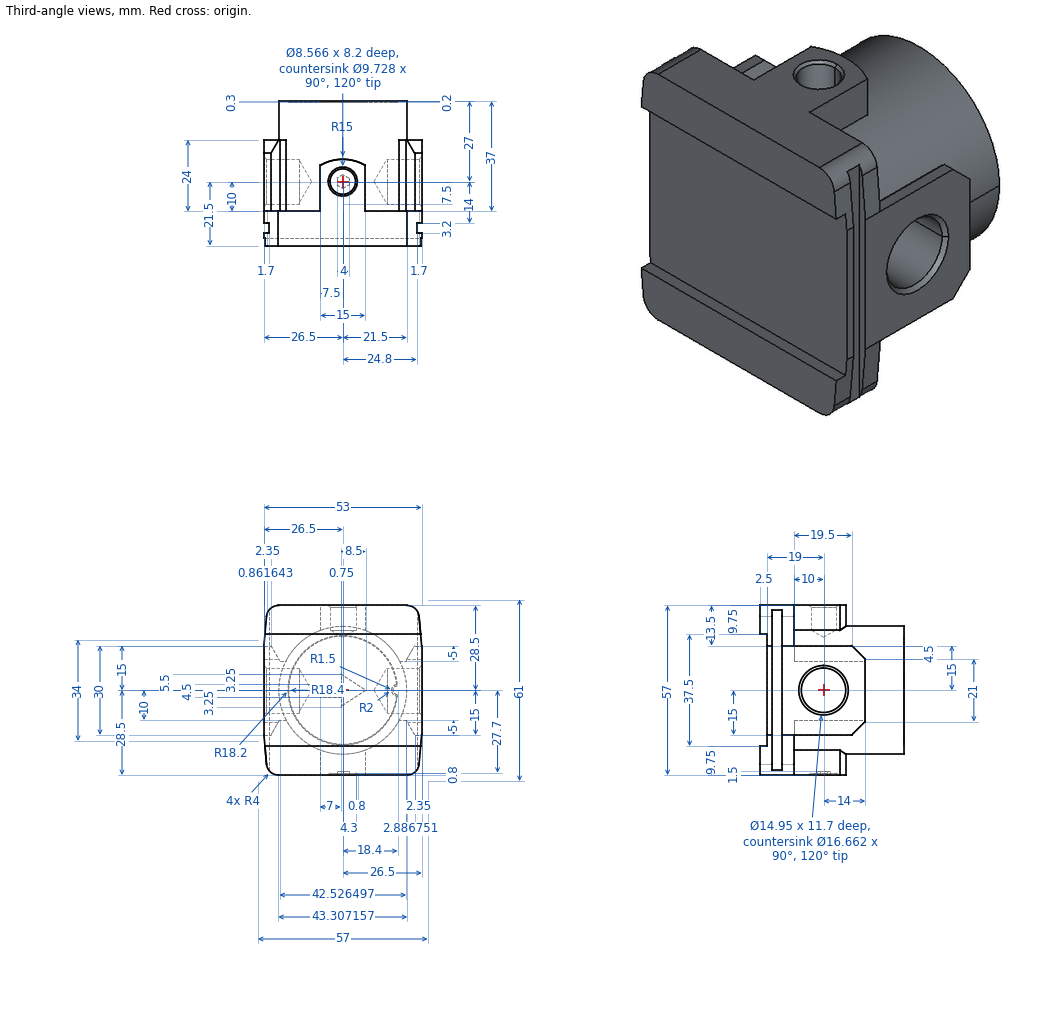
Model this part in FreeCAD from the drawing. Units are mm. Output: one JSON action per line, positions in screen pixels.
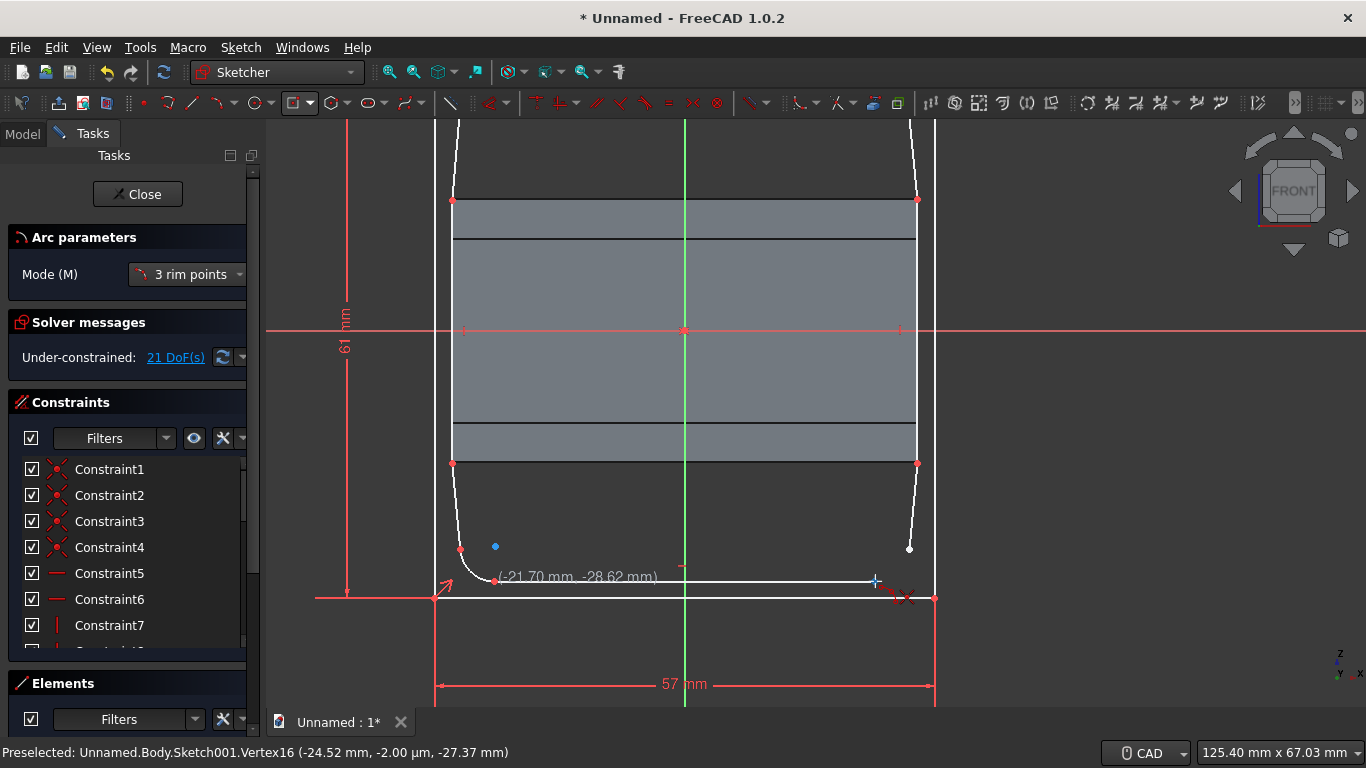
{"action": "left_click", "coordinate": [874, 582]}
{"action": "left_click", "coordinate": [909, 550]}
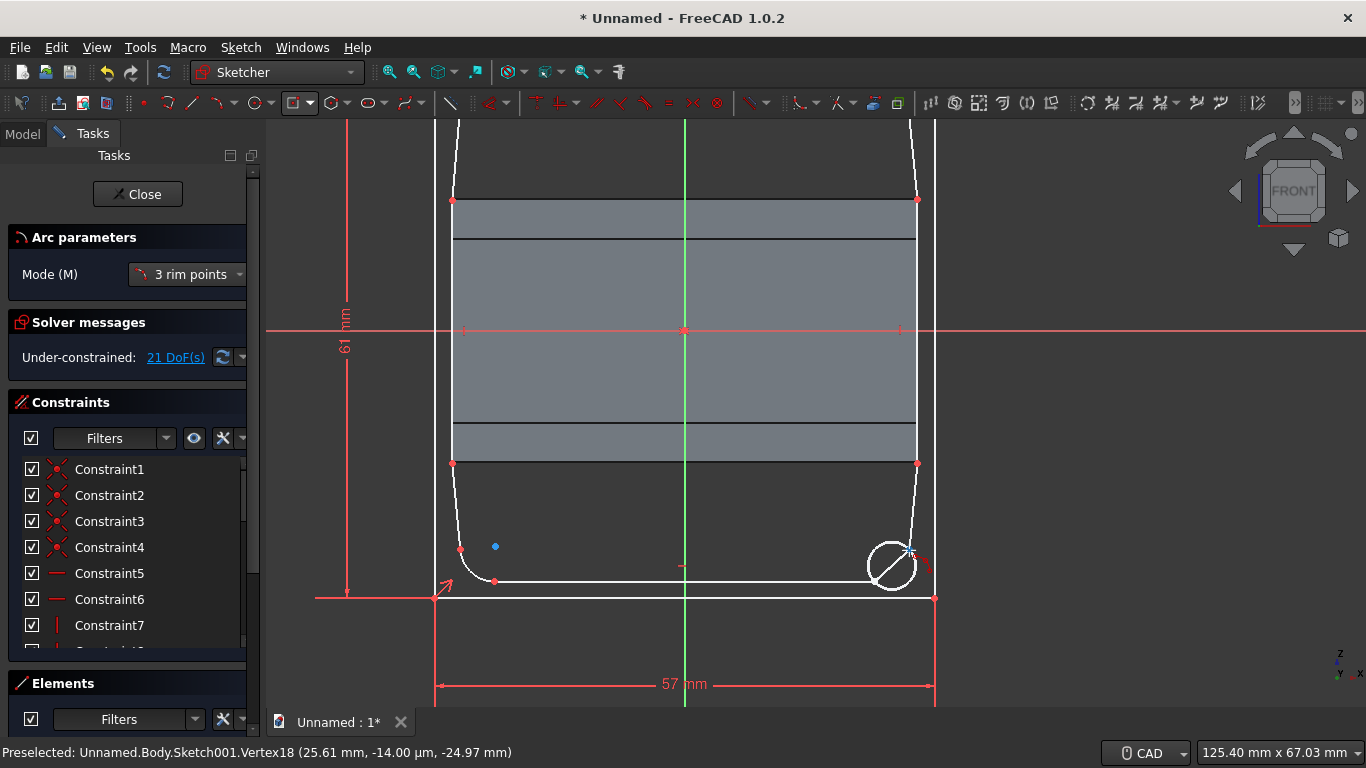
{"action": "scroll", "coordinate": [898, 572], "scroll_direction": "up", "scroll_amount": 3}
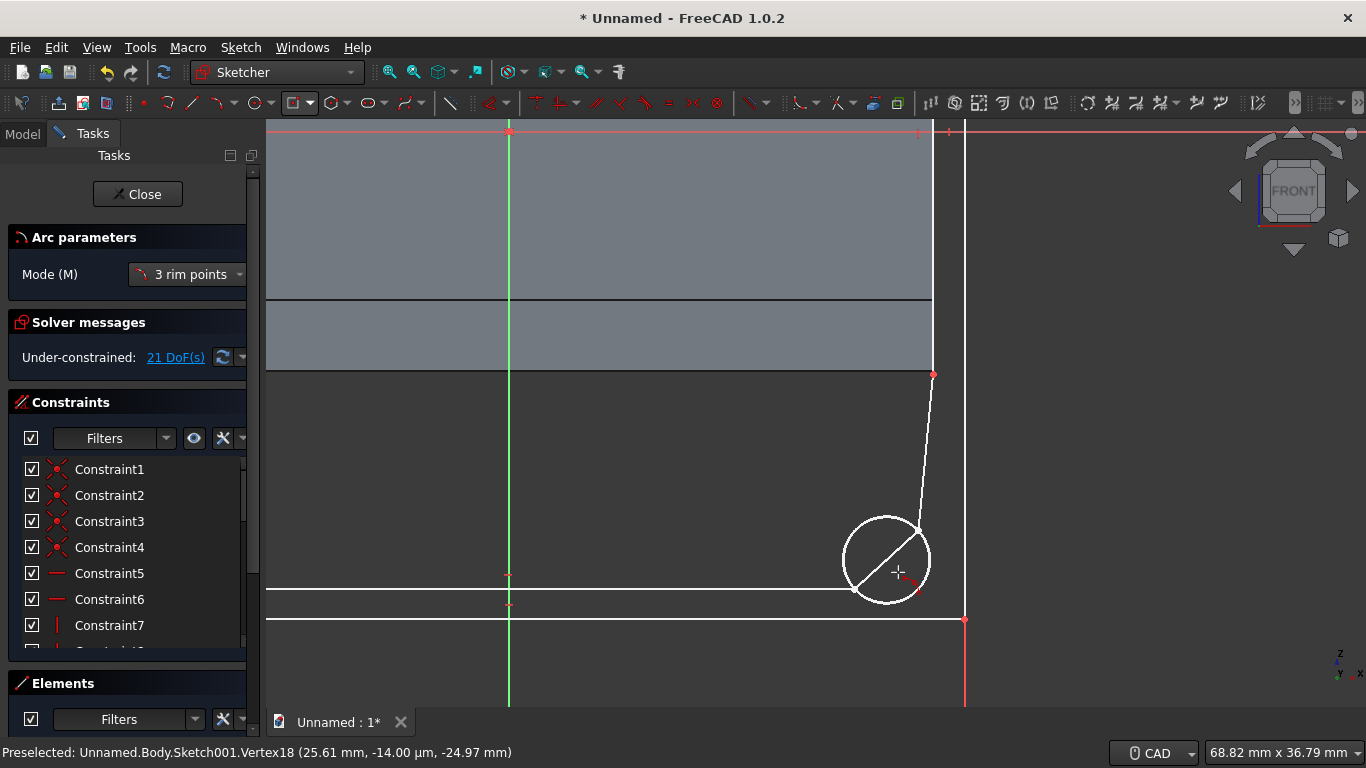
{"action": "left_click", "coordinate": [898, 570]}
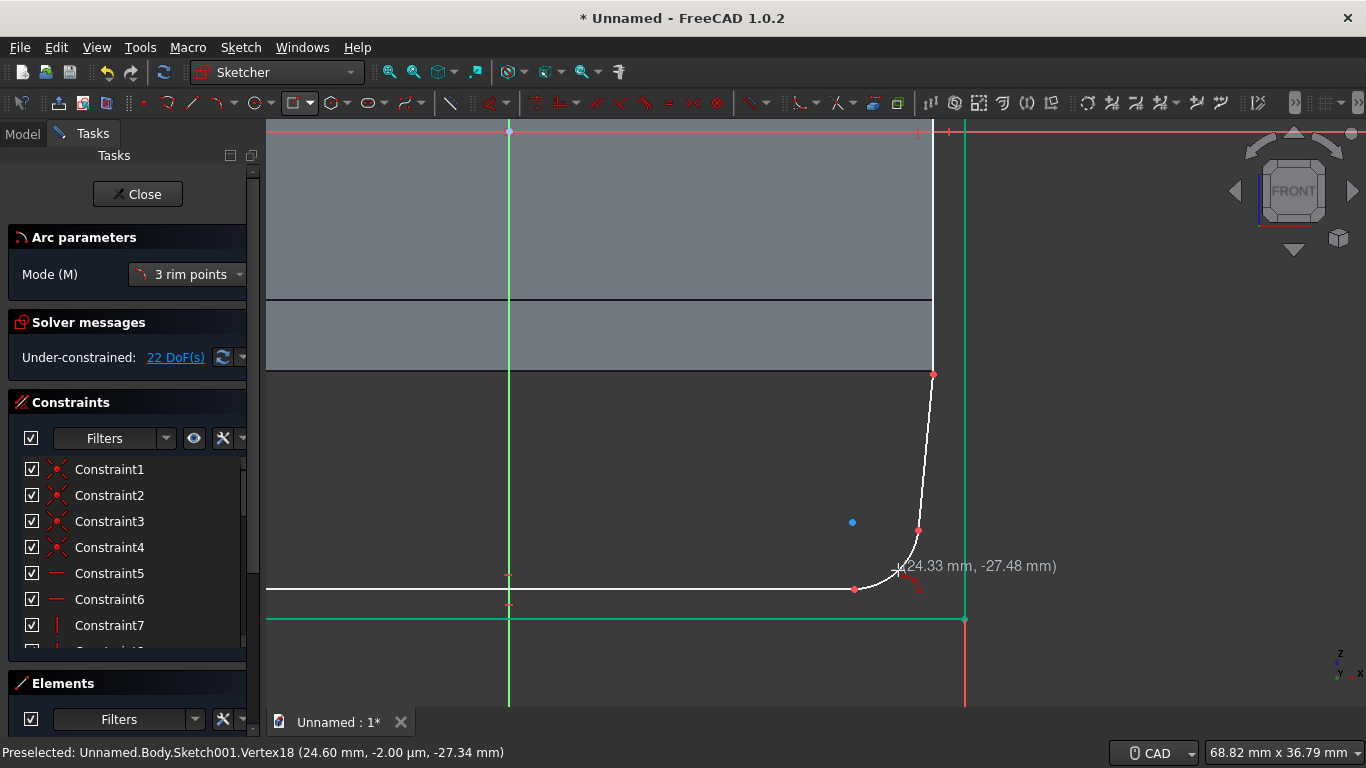
{"action": "scroll", "coordinate": [886, 577], "scroll_direction": "down", "scroll_amount": 5}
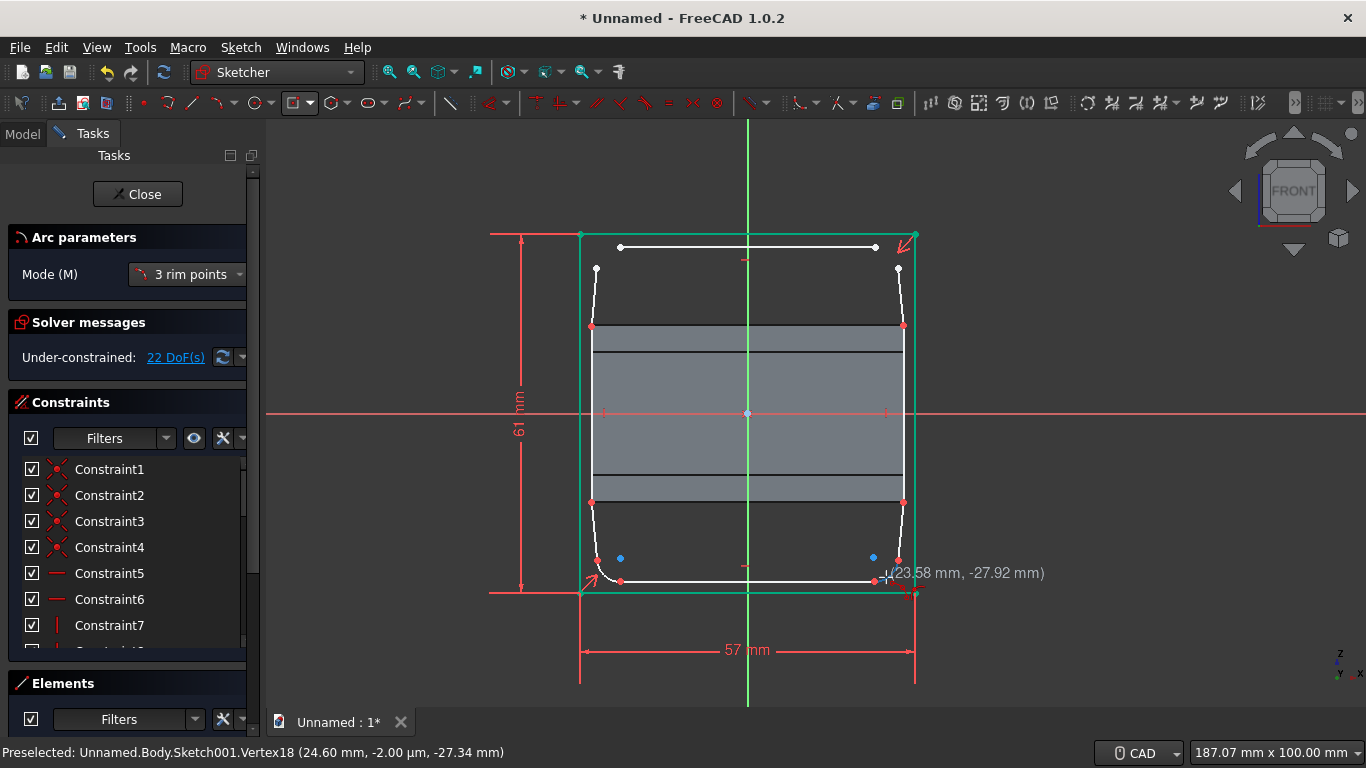
{"action": "left_click", "coordinate": [898, 268]}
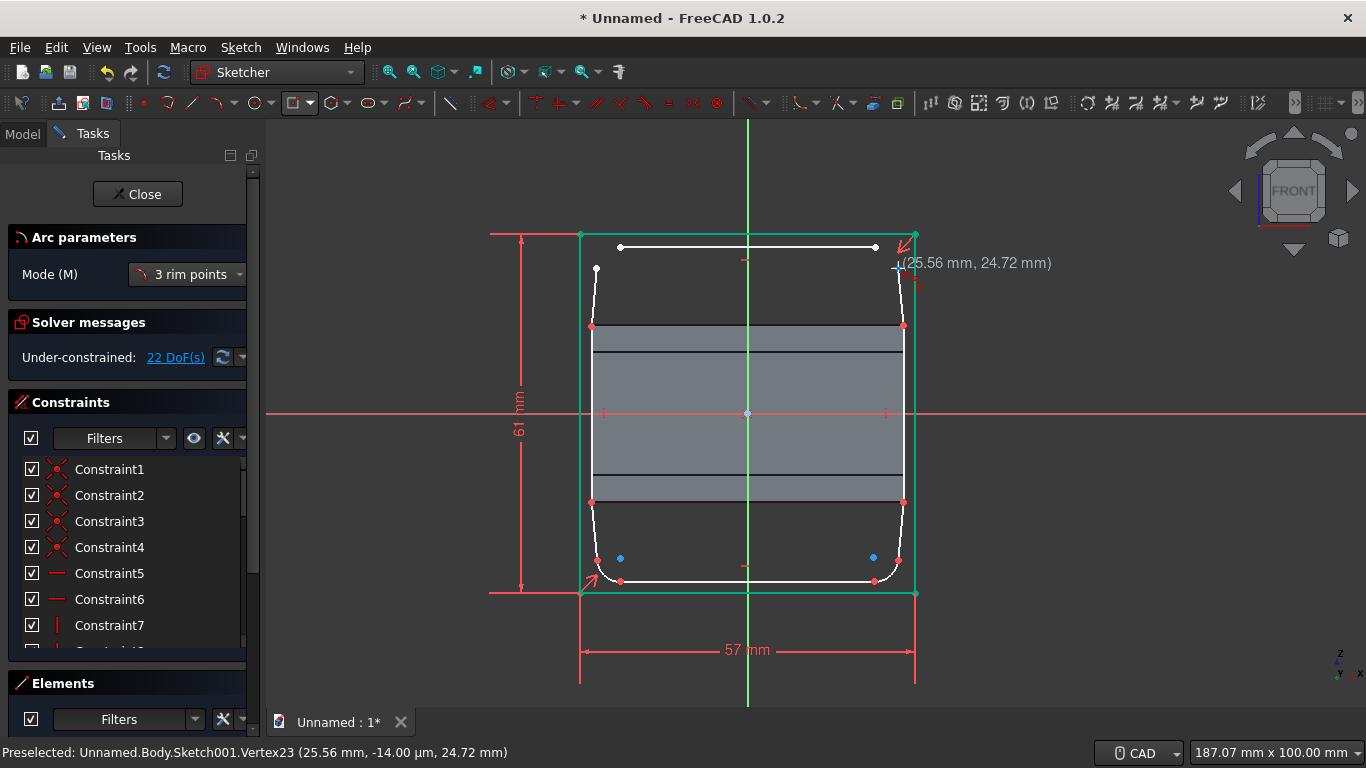
{"action": "scroll", "coordinate": [875, 246], "scroll_direction": "up", "scroll_amount": 2}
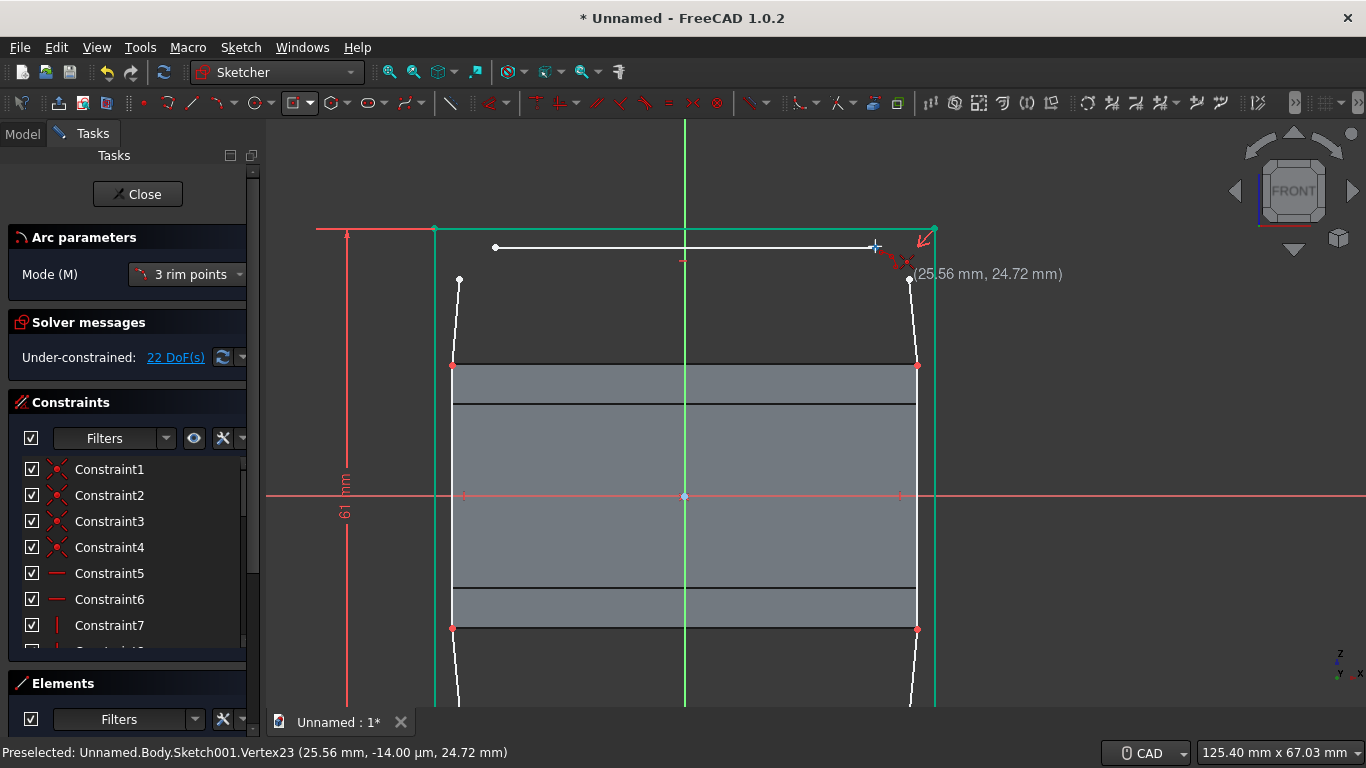
{"action": "left_click", "coordinate": [875, 248]}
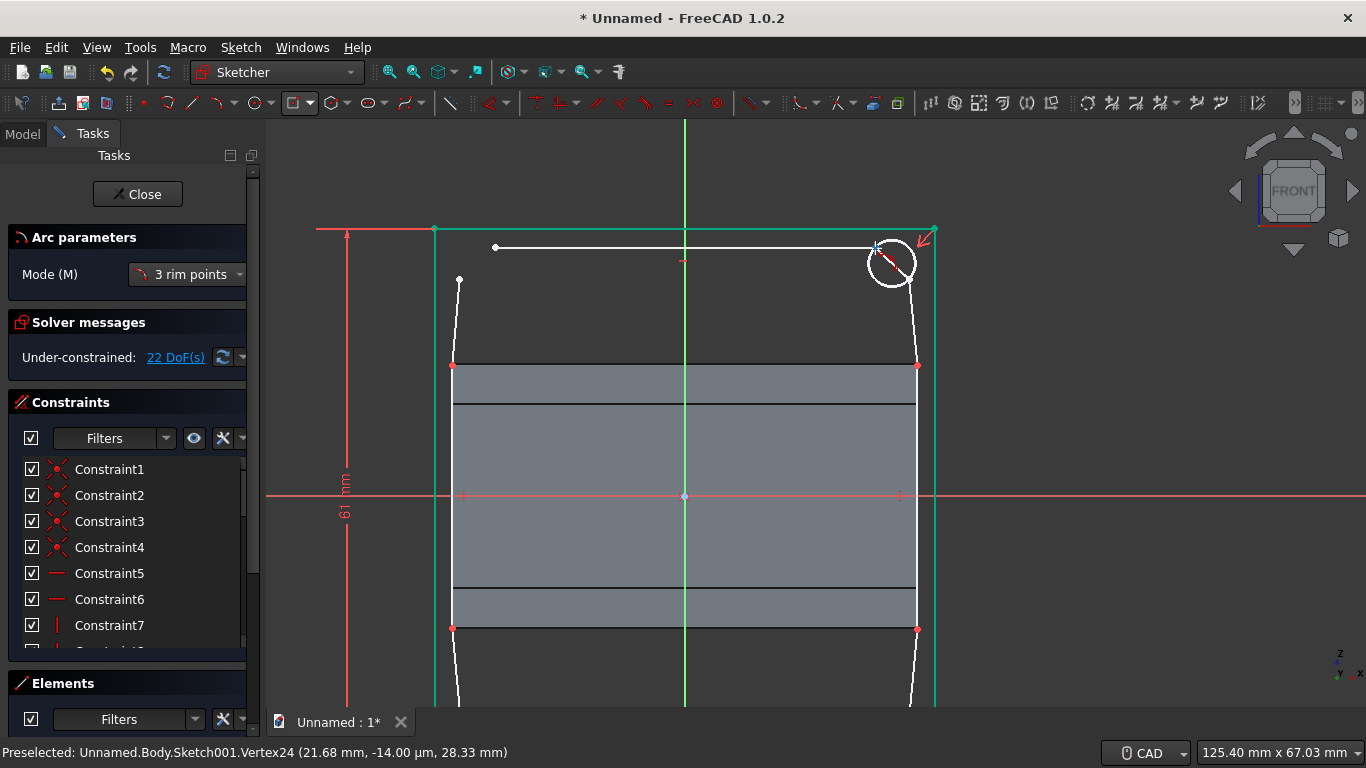
{"action": "scroll", "coordinate": [898, 255], "scroll_direction": "up", "scroll_amount": 3}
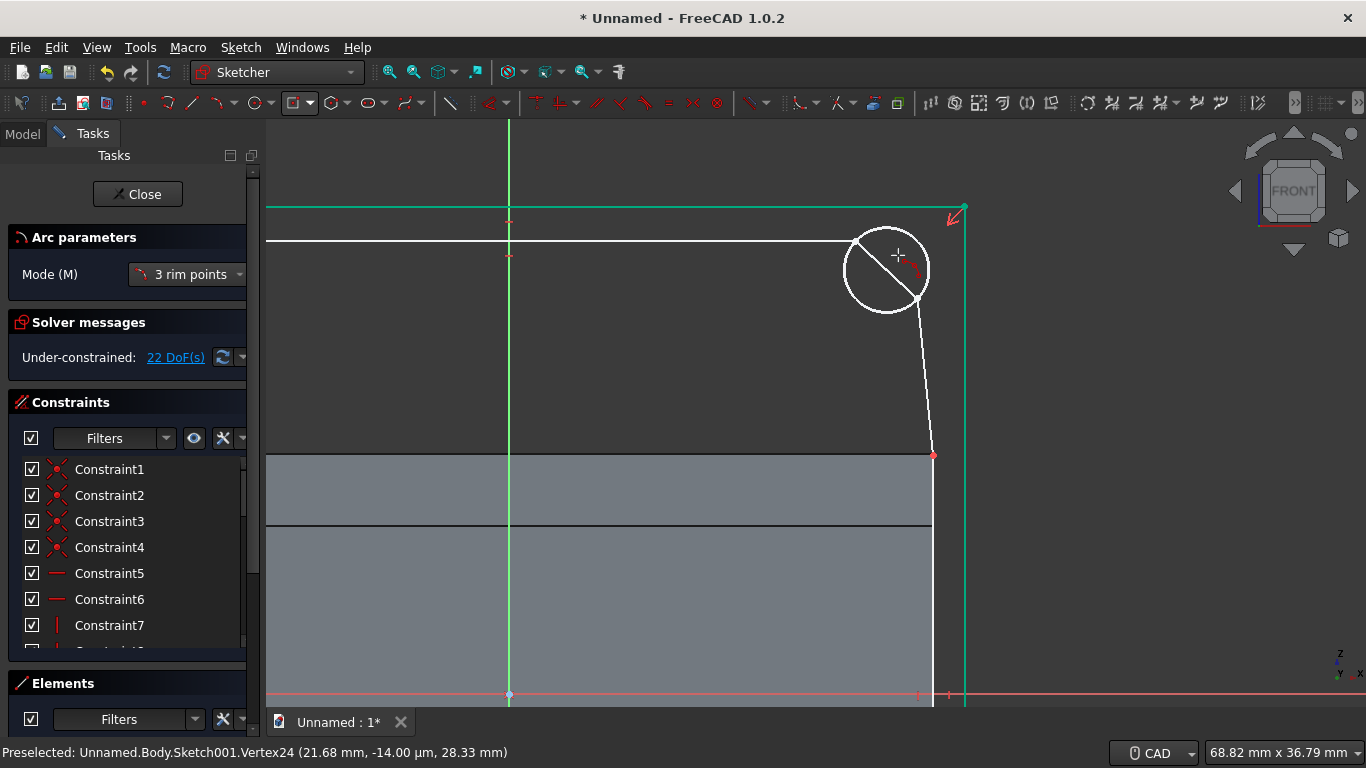
{"action": "left_click", "coordinate": [898, 255]}